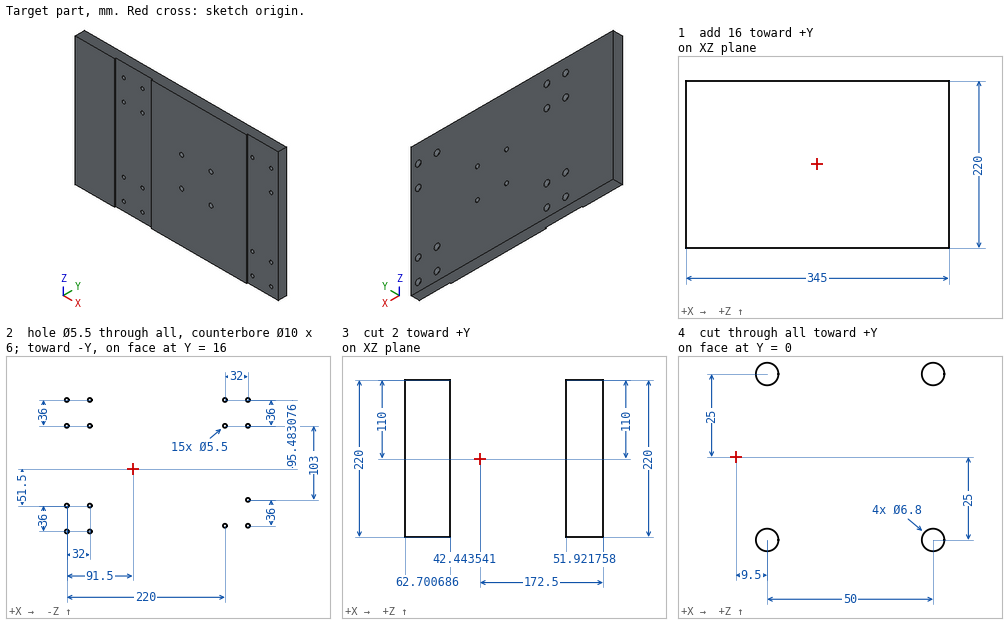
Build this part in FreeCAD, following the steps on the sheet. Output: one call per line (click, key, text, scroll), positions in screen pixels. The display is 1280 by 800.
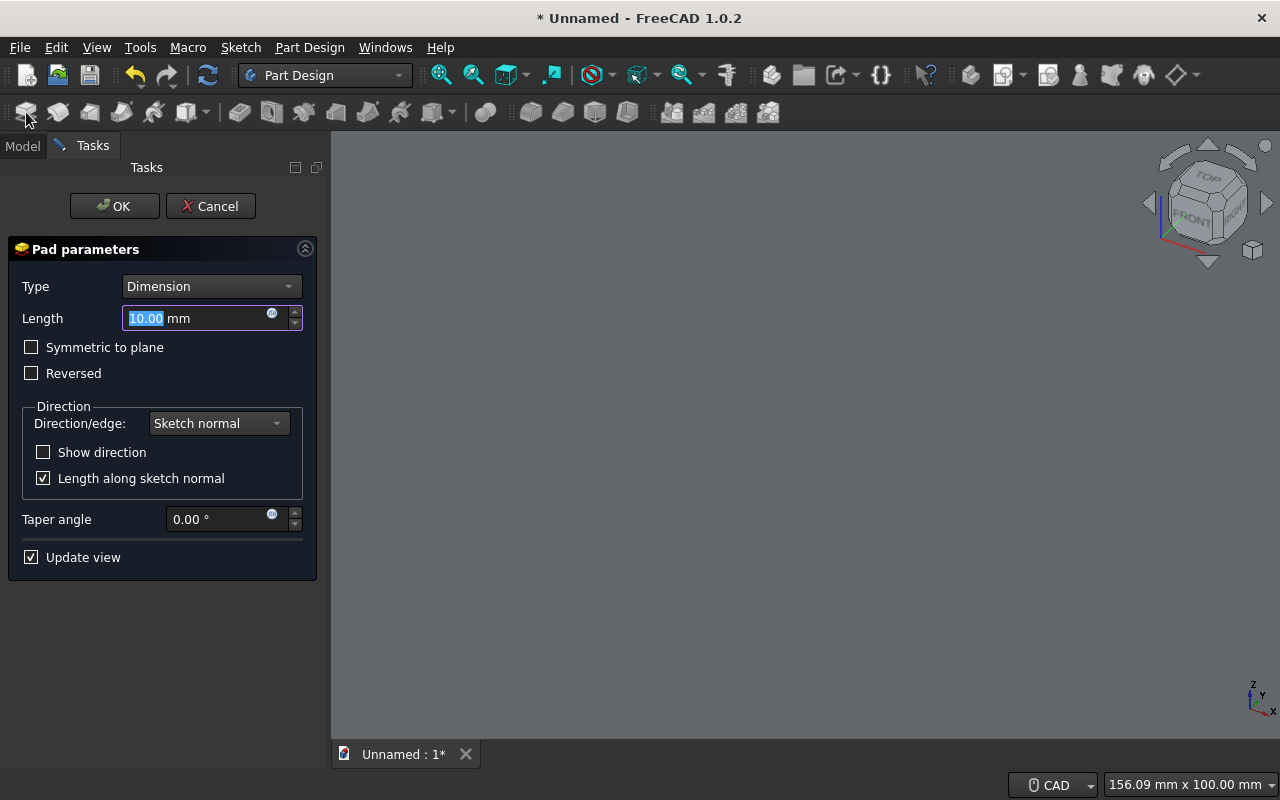
text(16)
key(Tab)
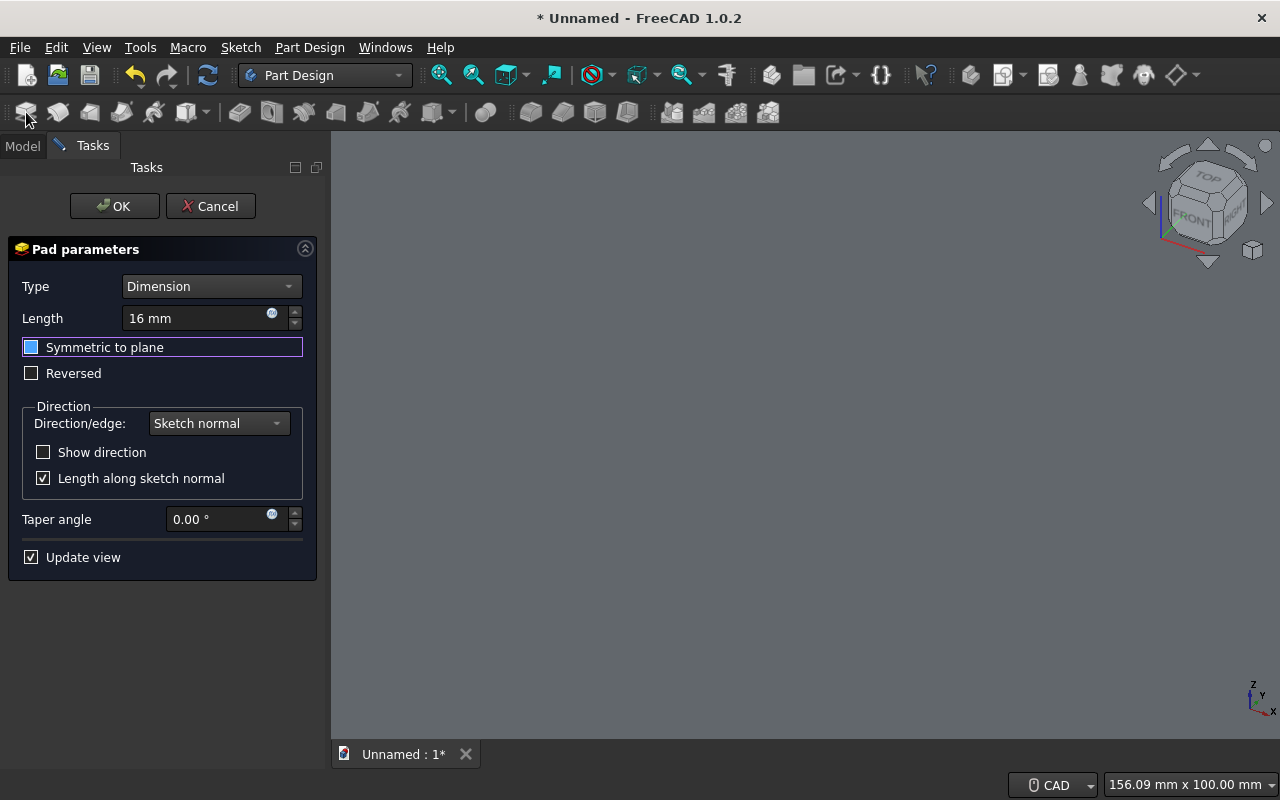
click(30, 373)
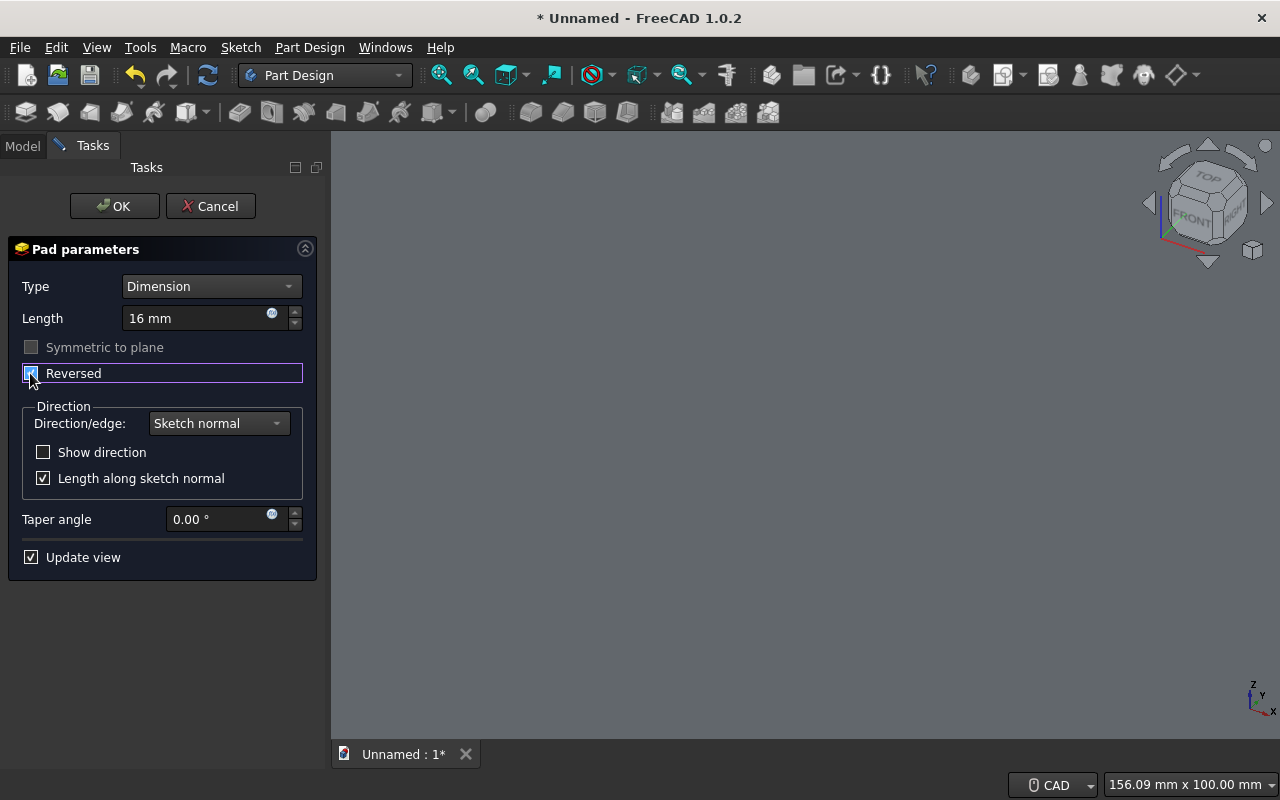
click(115, 206)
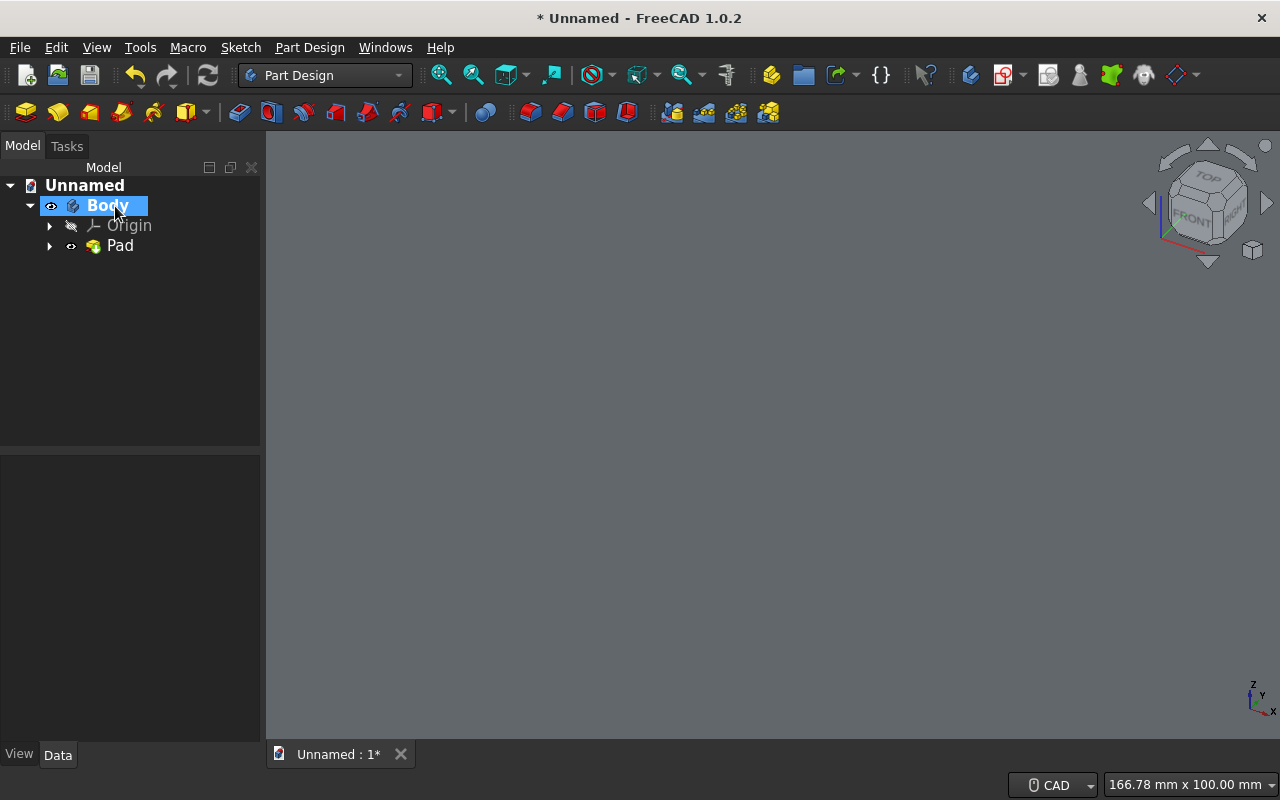
key(v)
key(f)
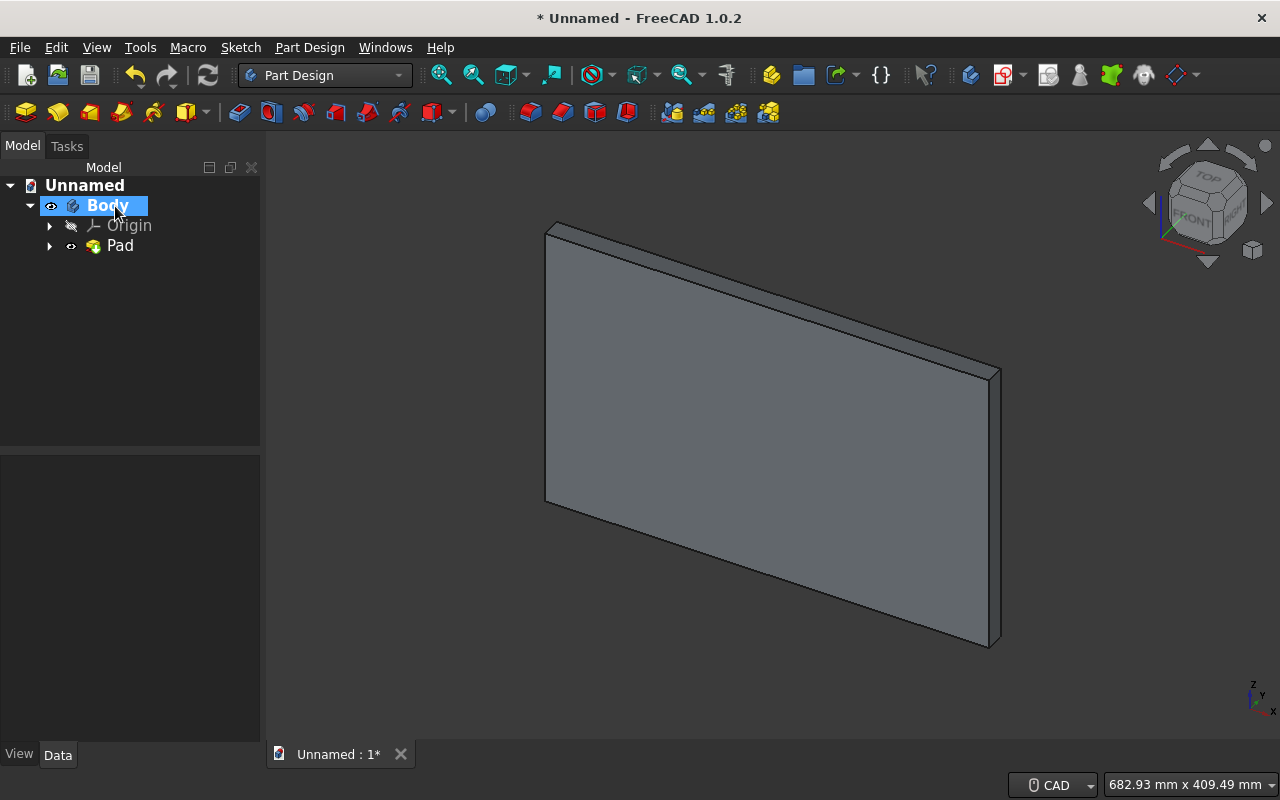
key(4)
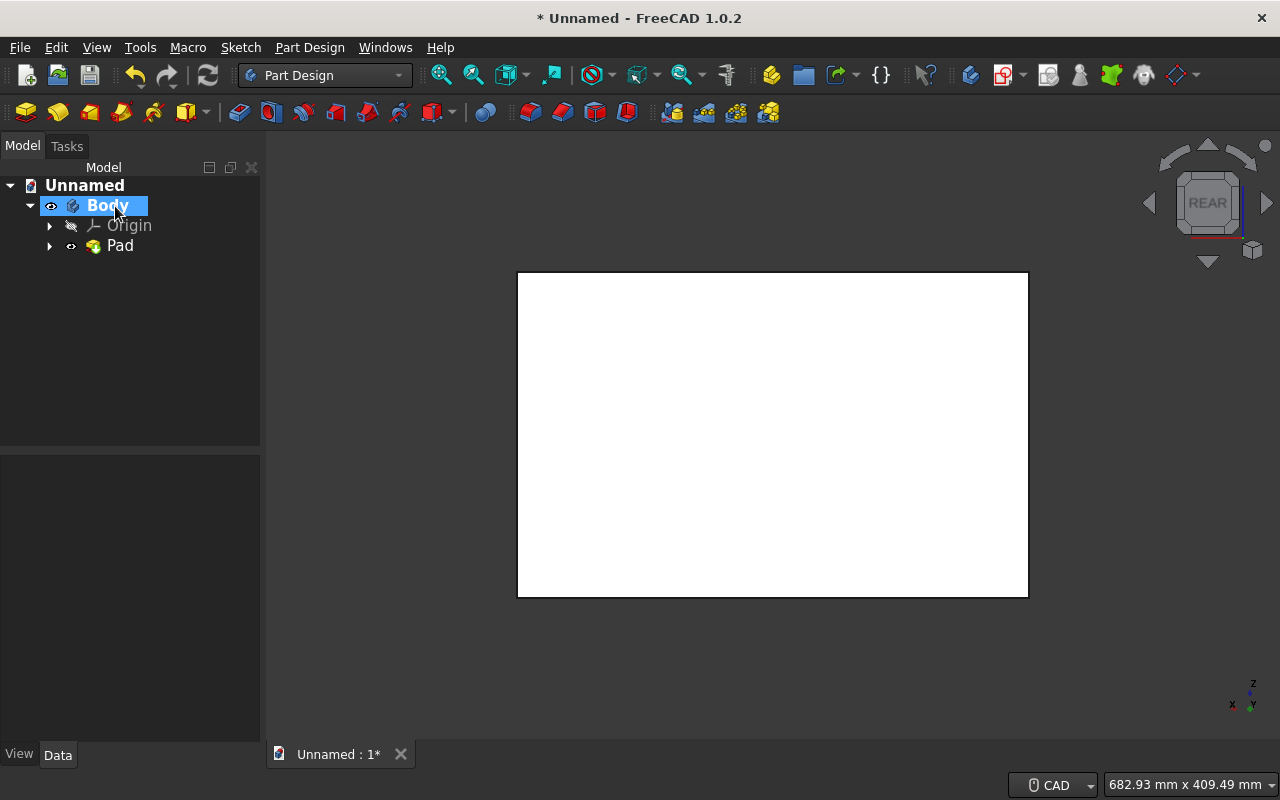
click(700, 434)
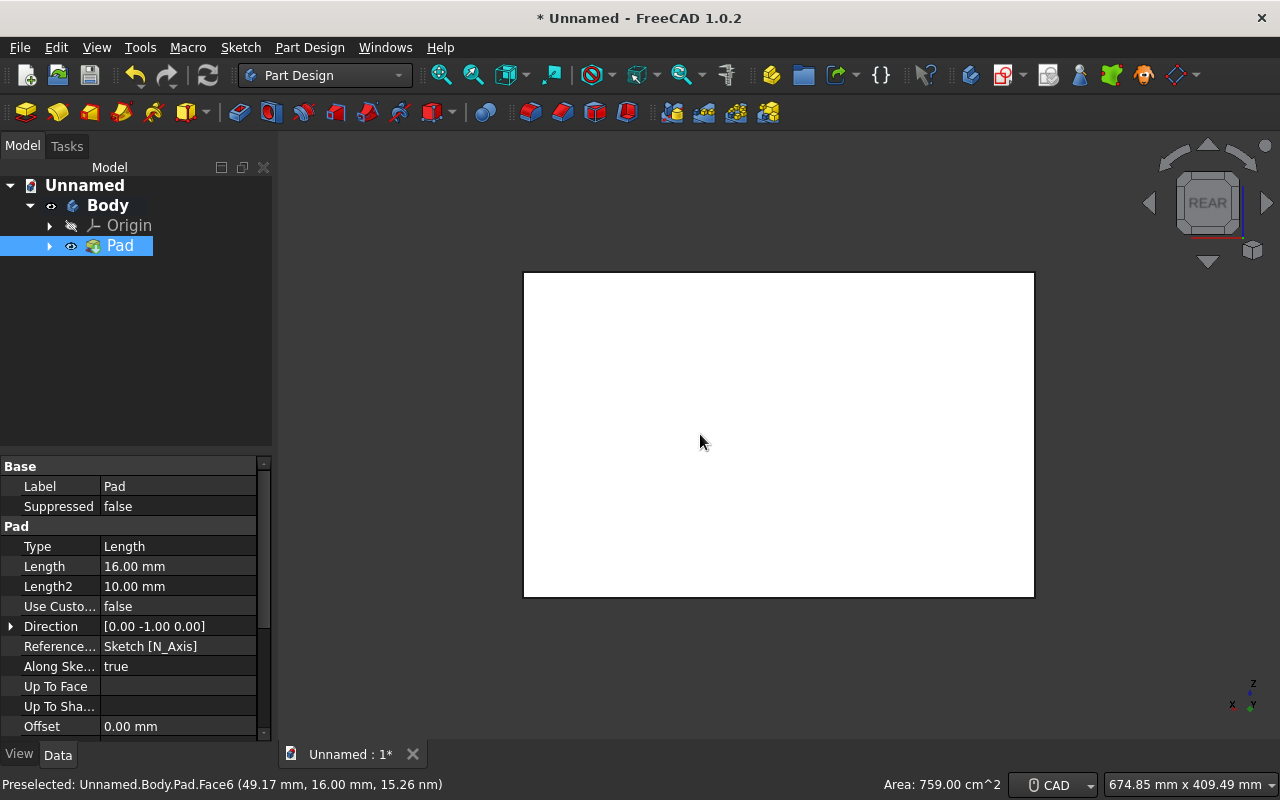
click(1004, 76)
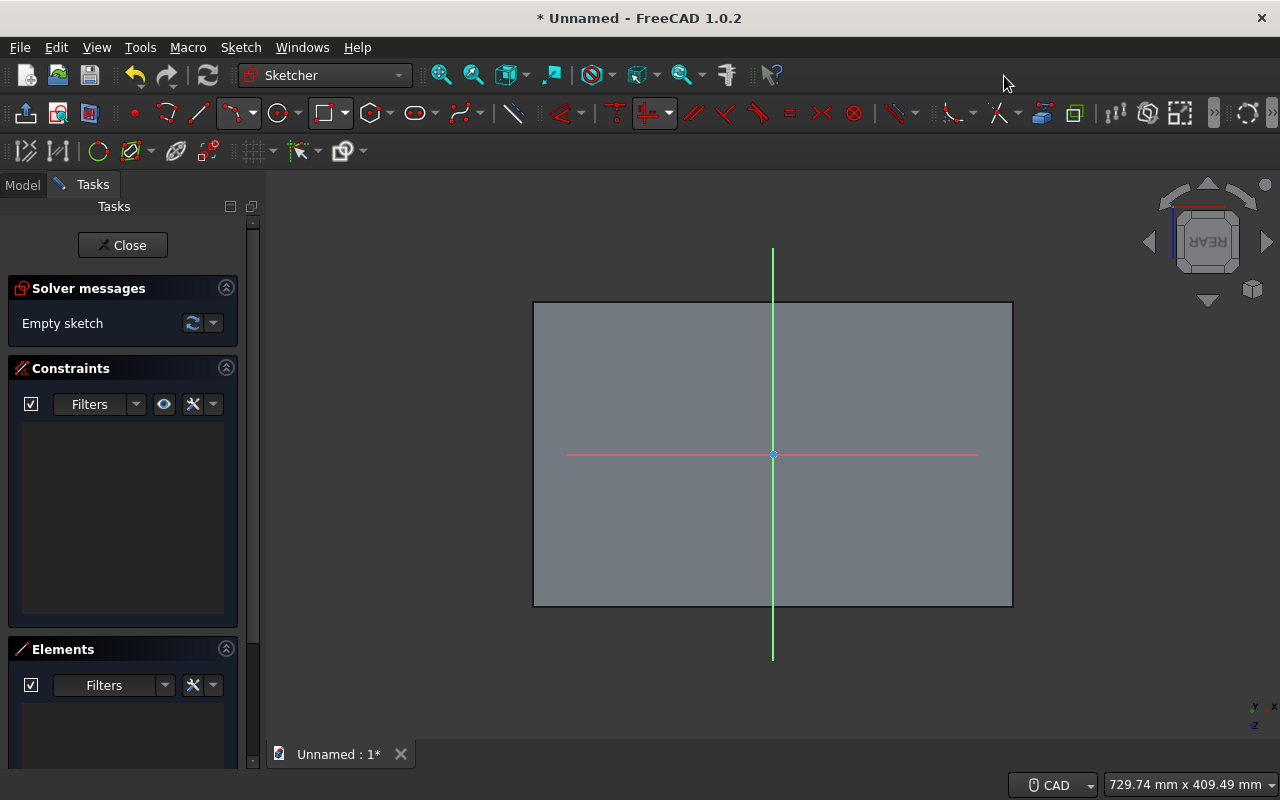
scroll(1058, 438, up, 2)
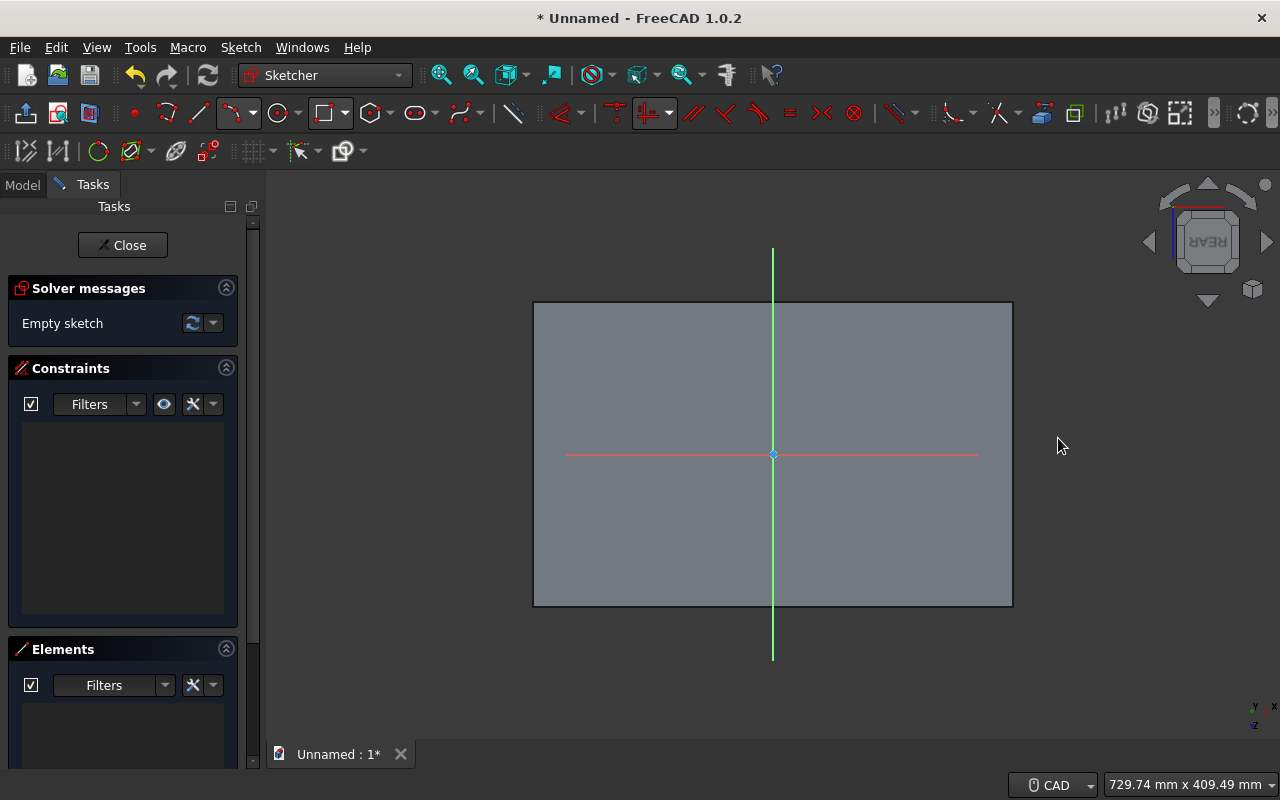
click(278, 114)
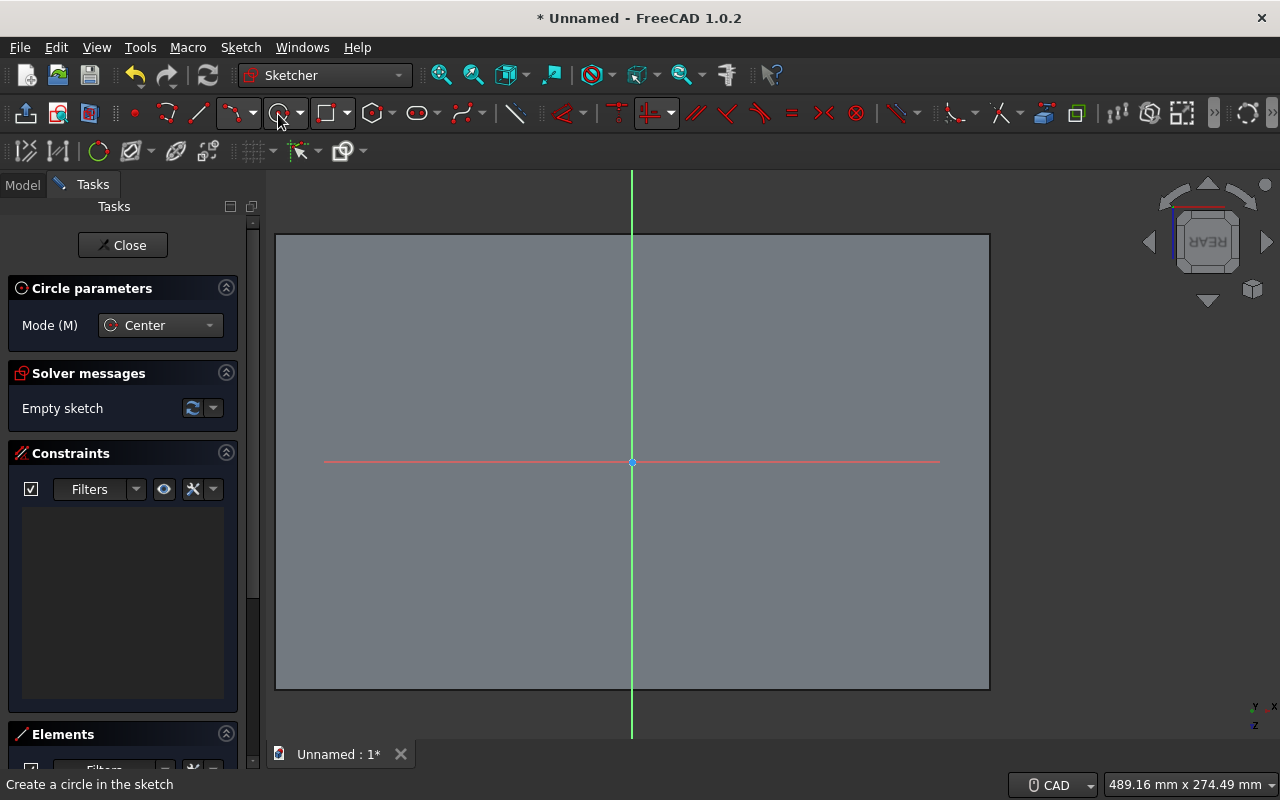
scroll(965, 264, up, 7)